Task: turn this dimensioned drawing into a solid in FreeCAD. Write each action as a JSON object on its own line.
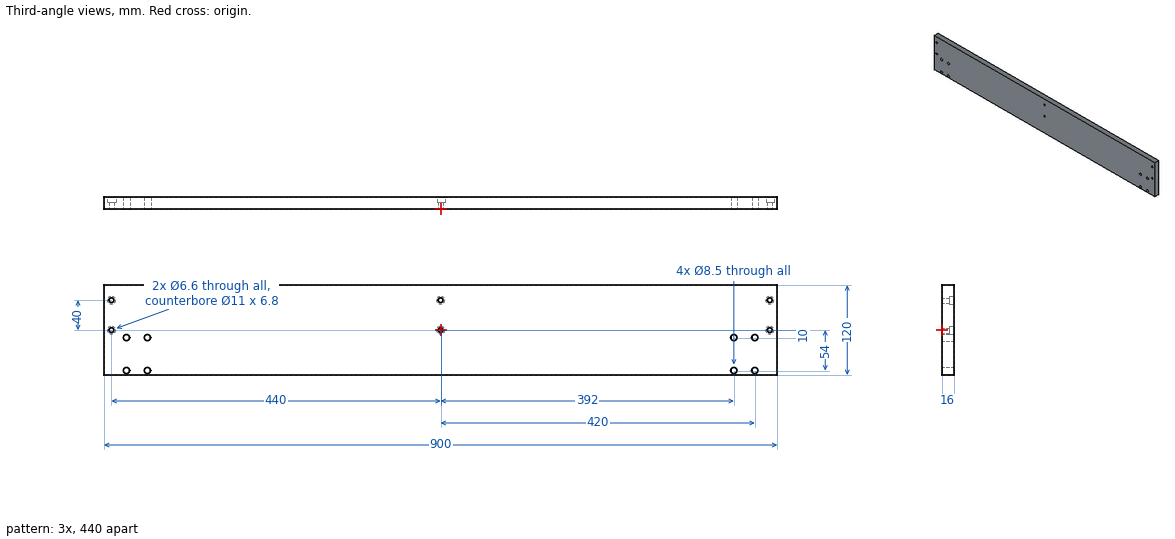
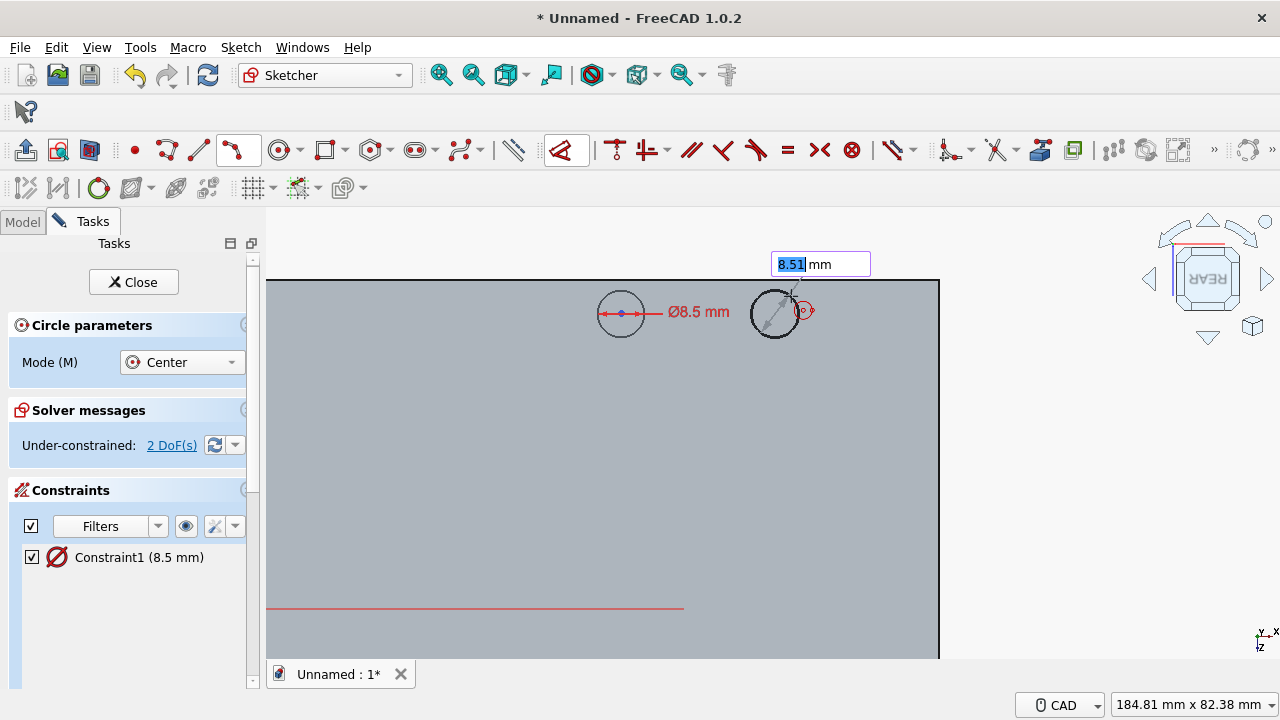
{"action": "type", "text": "8.5"}
{"action": "key", "text": "Return"}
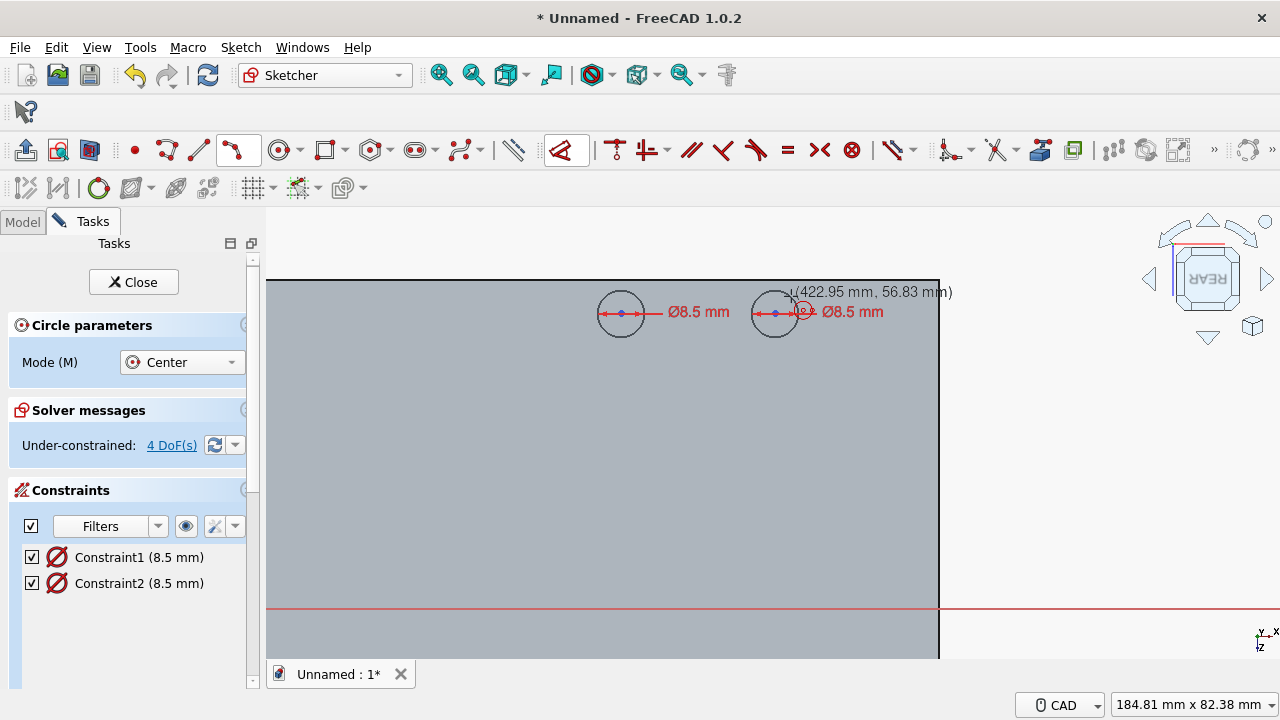
{"action": "left_click", "coordinate": [621, 554]}
{"action": "mouse_move", "coordinate": [638, 537]}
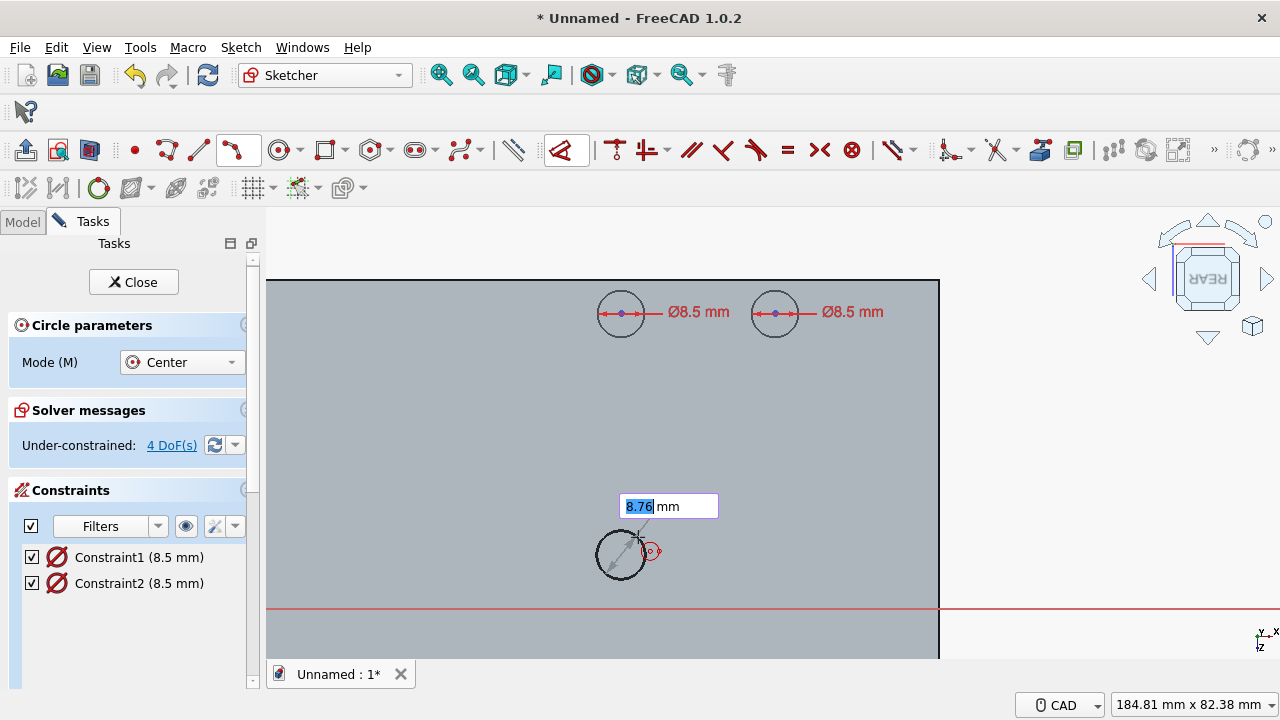
{"action": "type", "text": "8.5"}
{"action": "key", "text": "Return"}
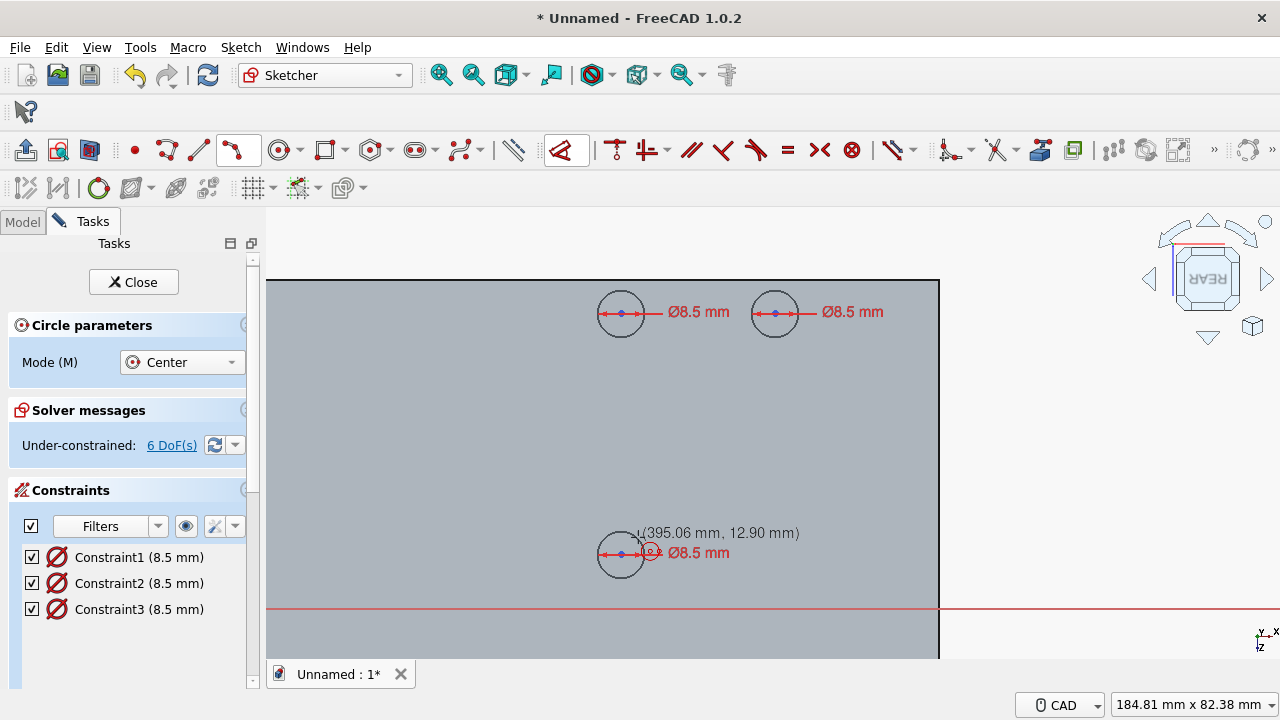
{"action": "left_click", "coordinate": [775, 554]}
{"action": "mouse_move", "coordinate": [791, 537]}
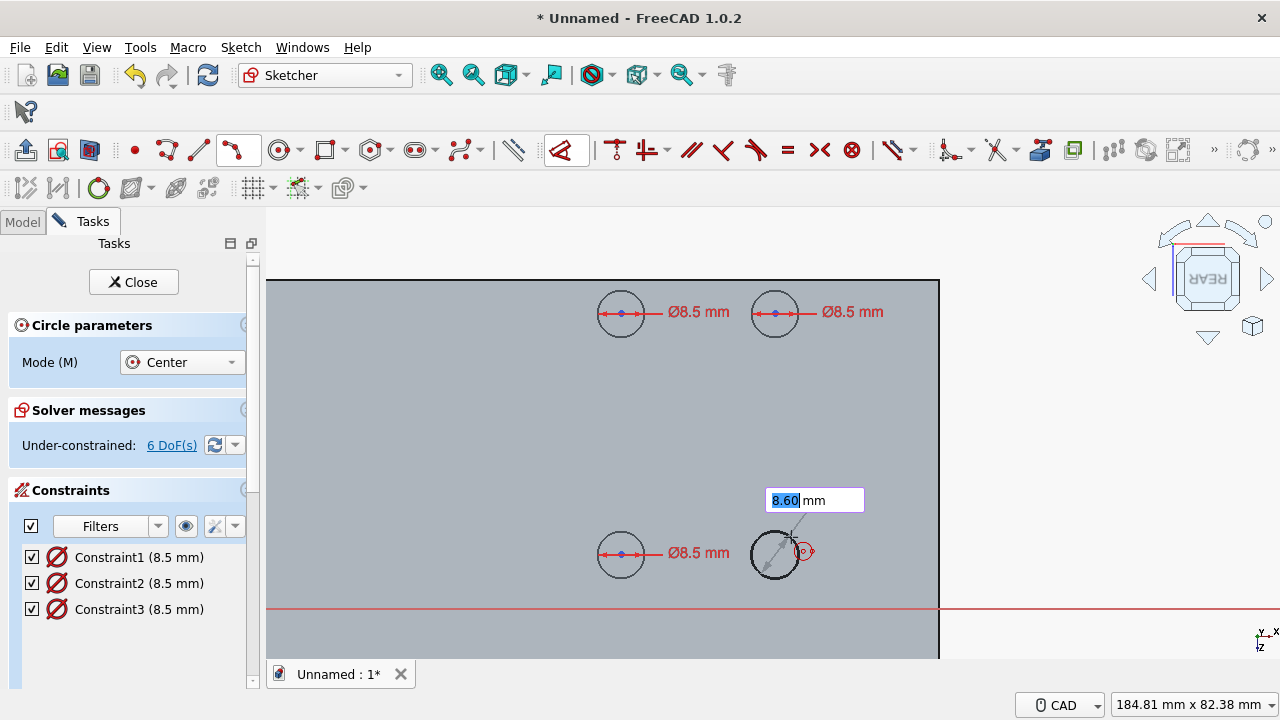
{"action": "type", "text": "8.5"}
{"action": "key", "text": "Return"}
{"action": "key", "text": "Escape"}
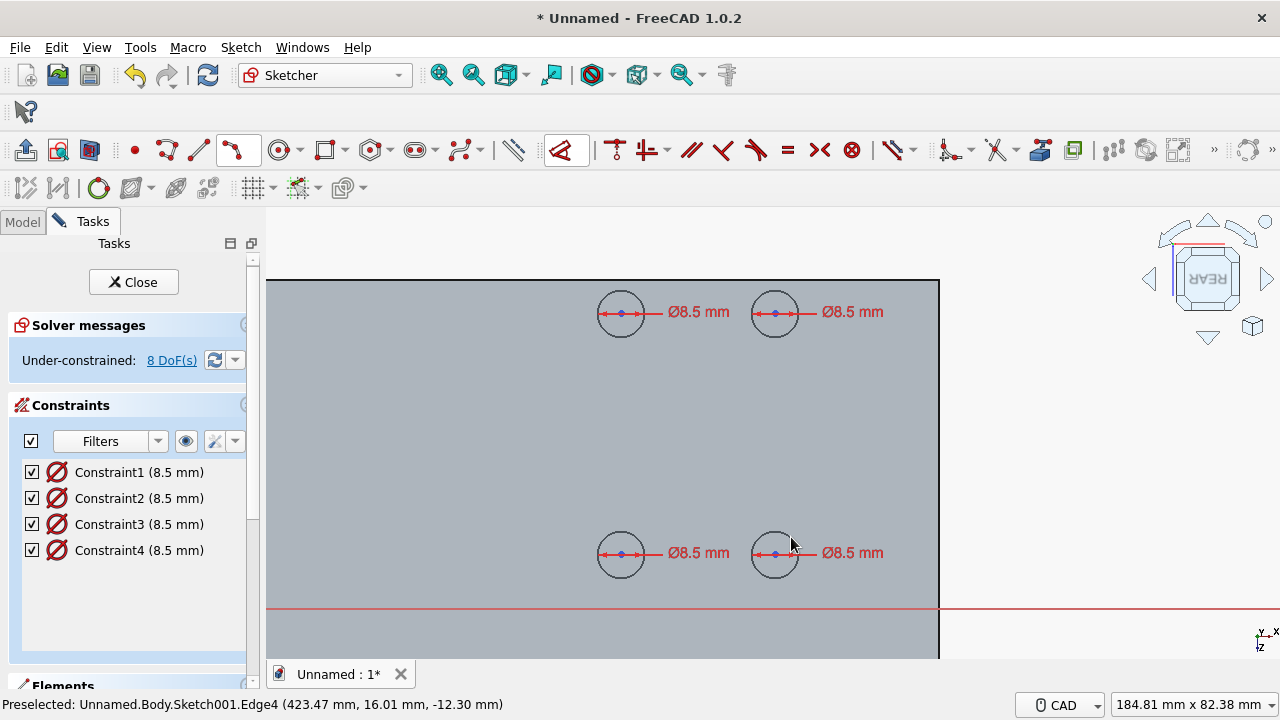
{"action": "left_click", "coordinate": [621, 314]}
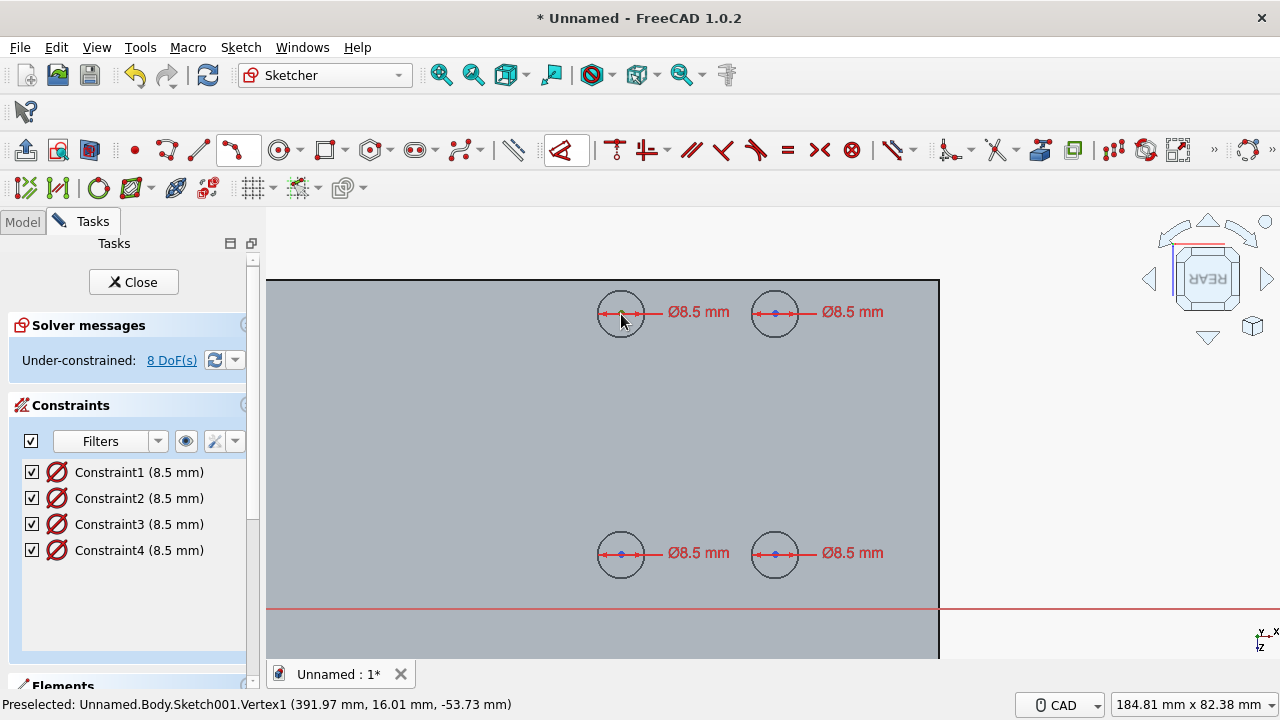
{"action": "key", "text": "i"}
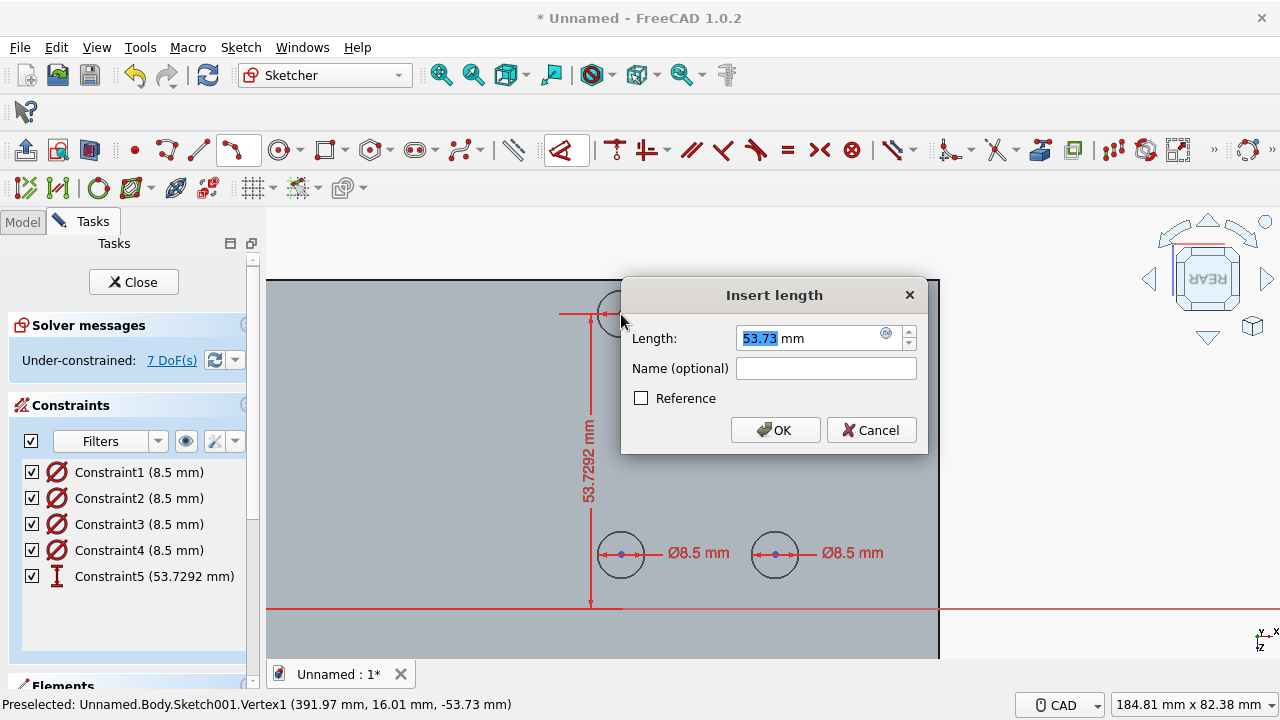
{"action": "type", "text": "54"}
{"action": "key", "text": "Return"}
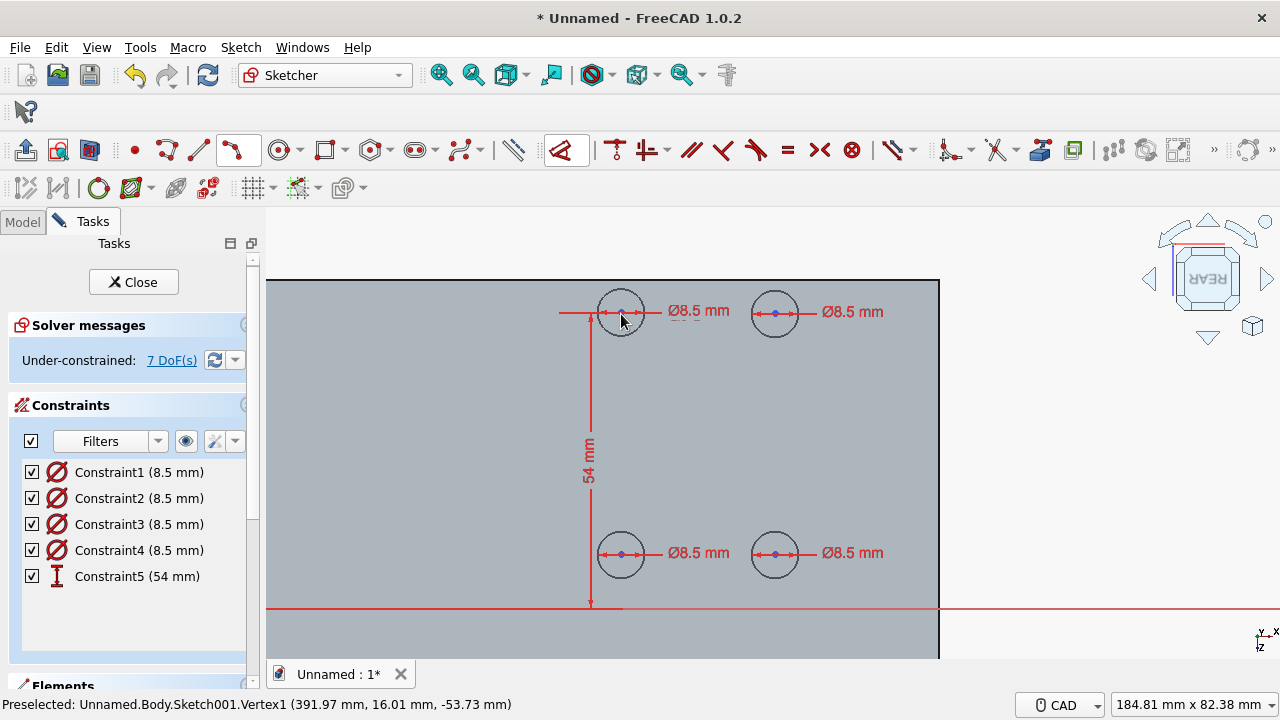
{"action": "left_click", "coordinate": [775, 314]}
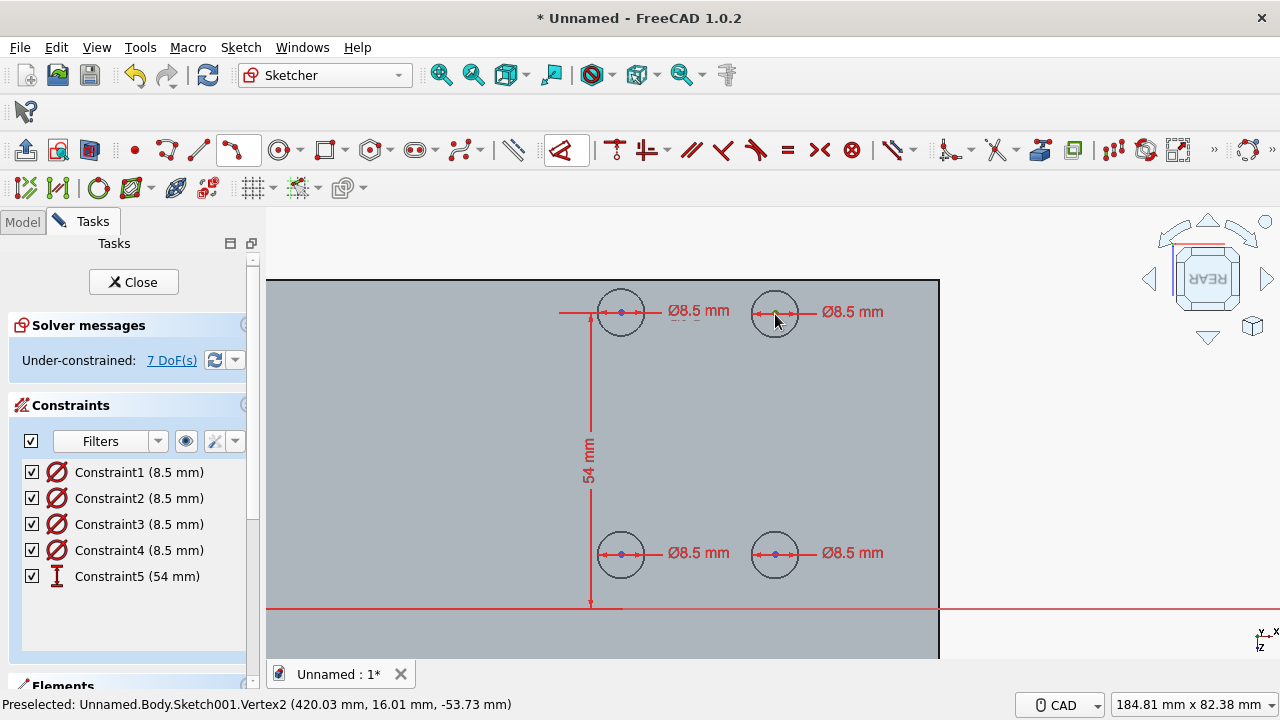
{"action": "key", "text": "i"}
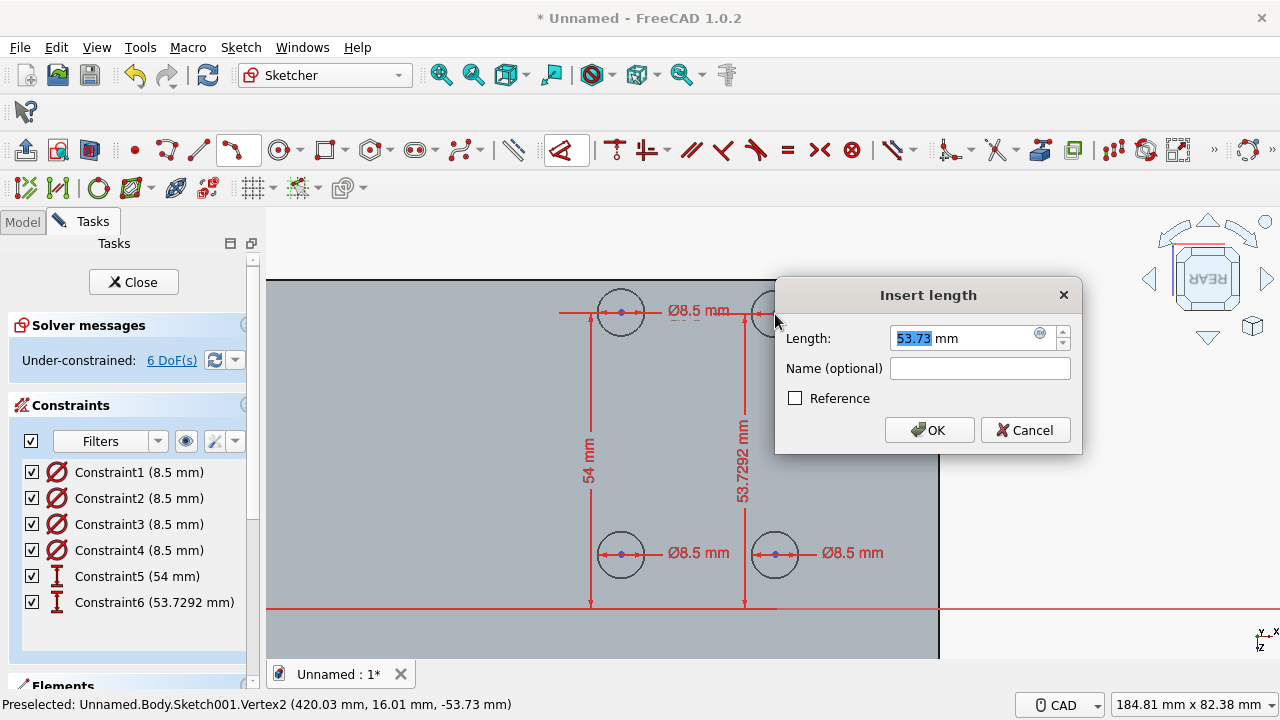
{"action": "type", "text": "54"}
{"action": "key", "text": "Return"}